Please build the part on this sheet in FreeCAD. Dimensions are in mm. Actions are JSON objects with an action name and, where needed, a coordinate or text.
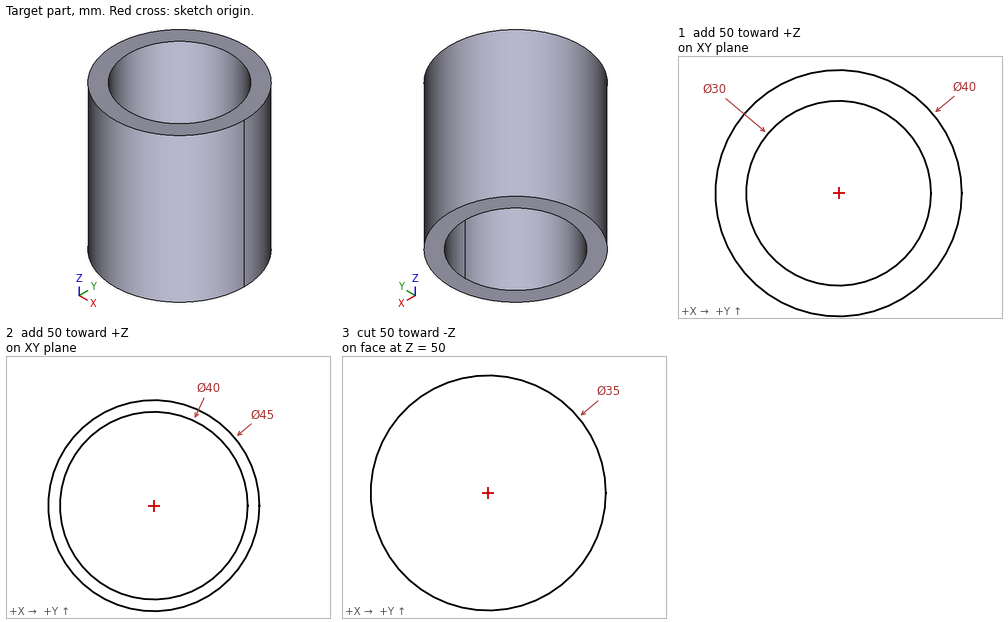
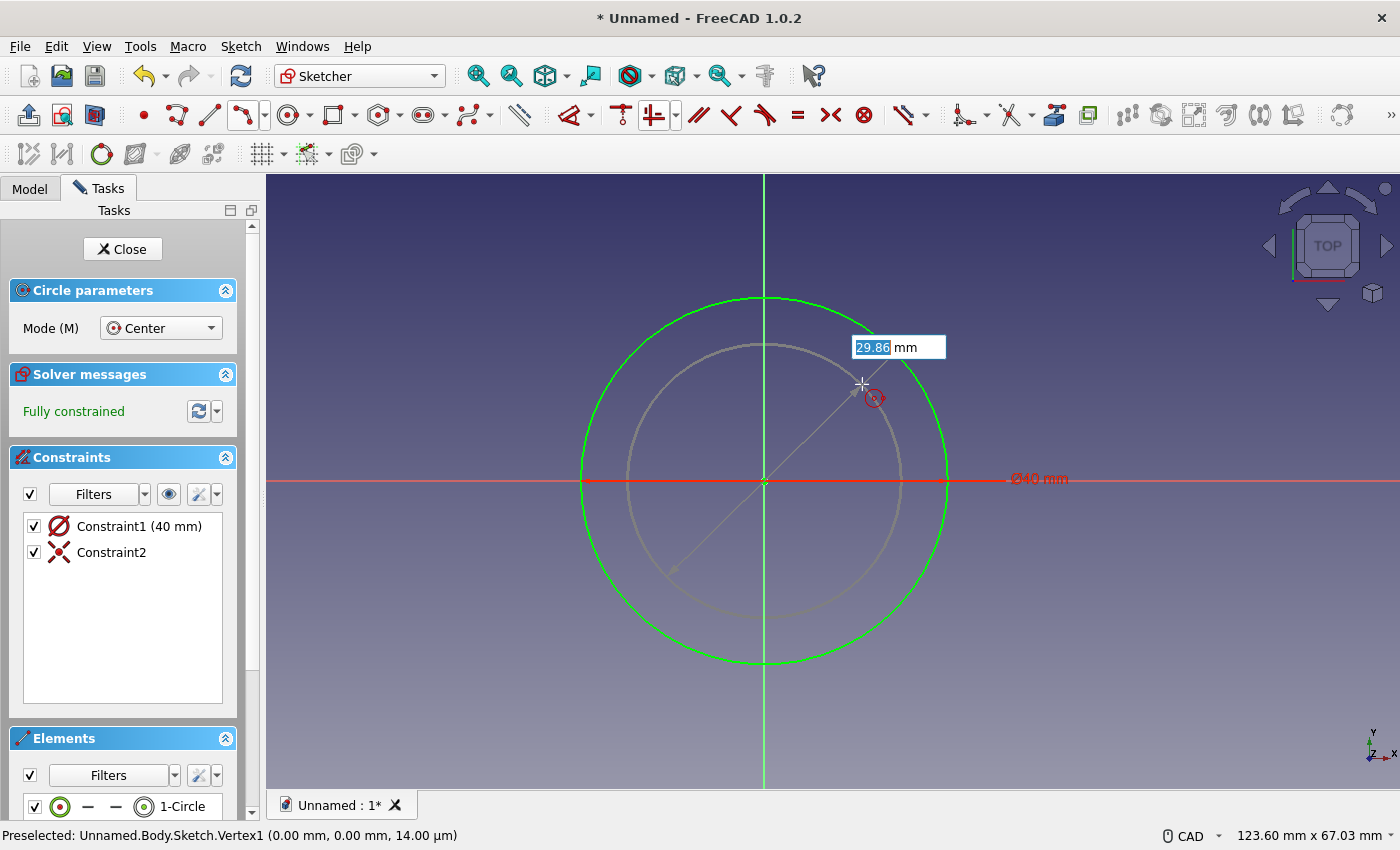
{"action": "type", "text": "30"}
{"action": "key", "text": "Return"}
{"action": "key", "text": "Escape"}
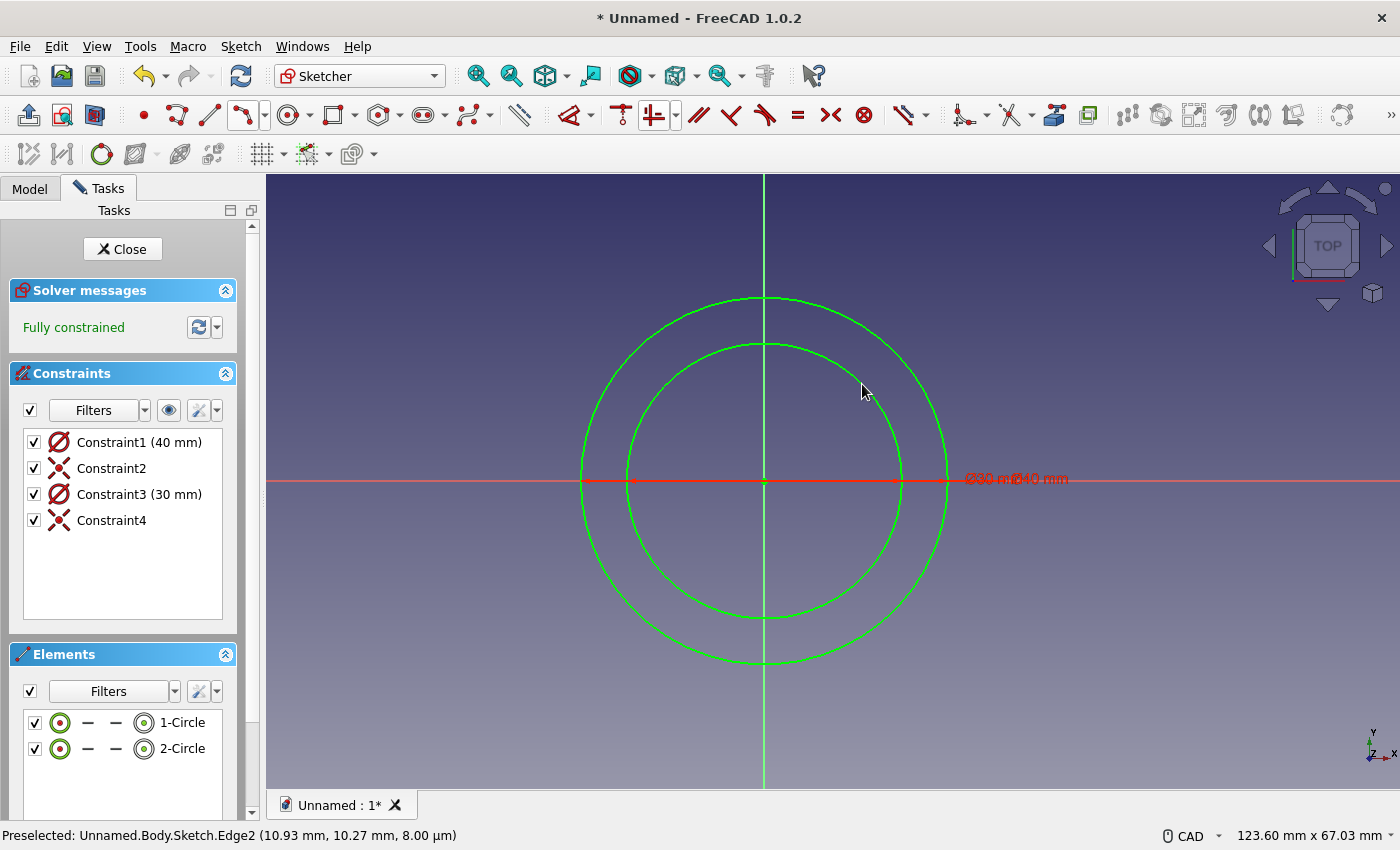
{"action": "left_click", "coordinate": [123, 249]}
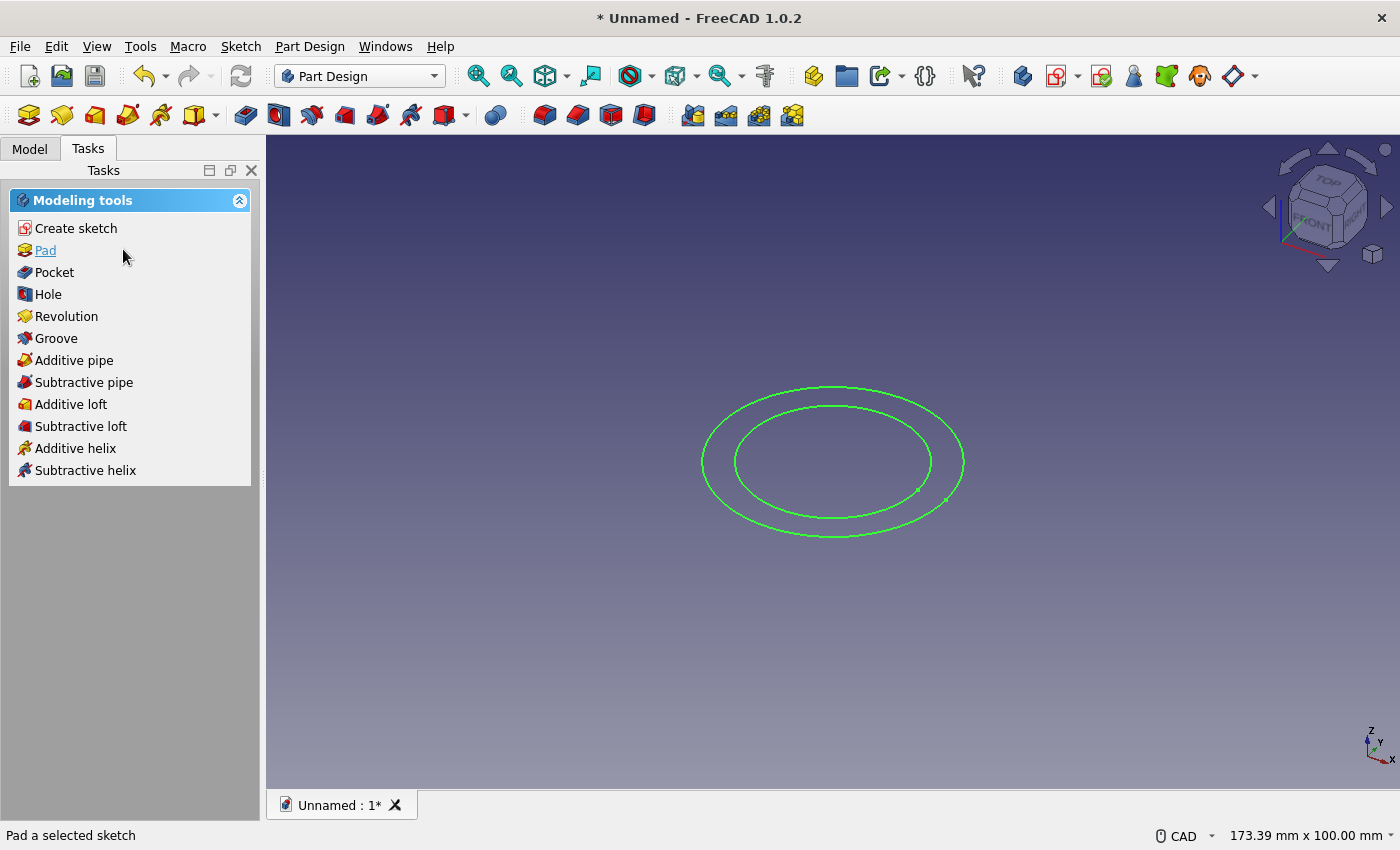
{"action": "left_click", "coordinate": [29, 116]}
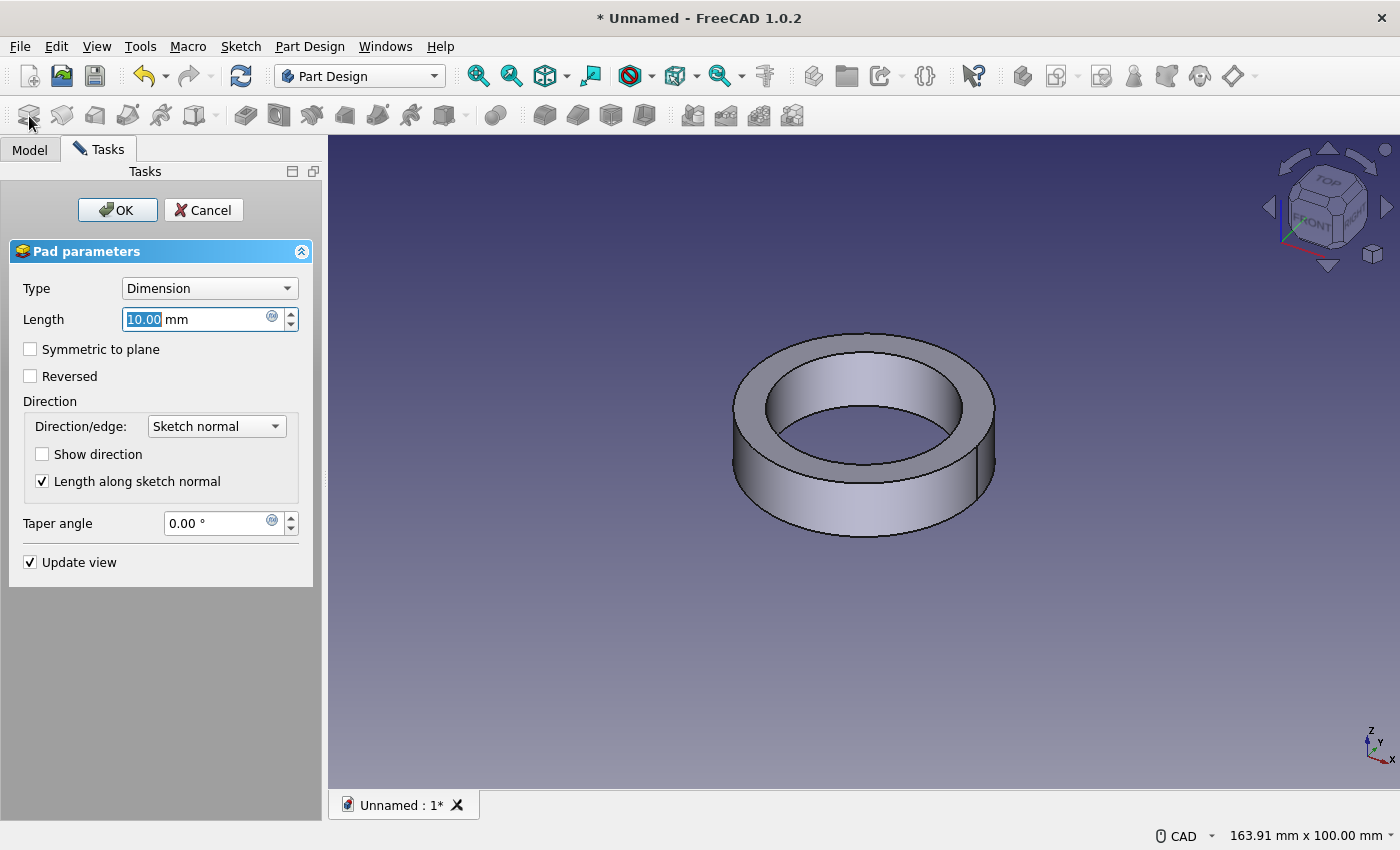
{"action": "type", "text": "50"}
{"action": "key", "text": "Tab"}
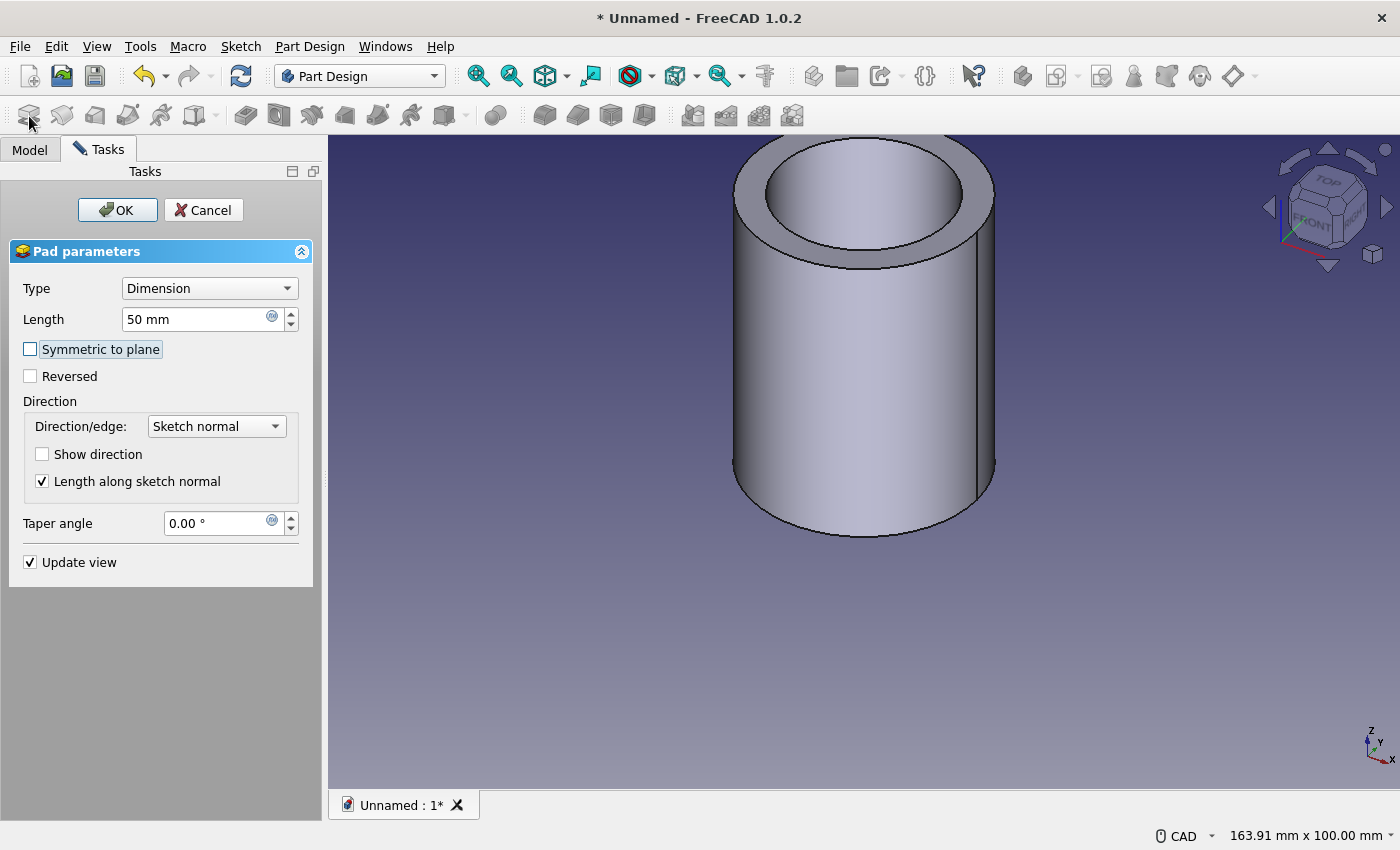
{"action": "left_click", "coordinate": [118, 210]}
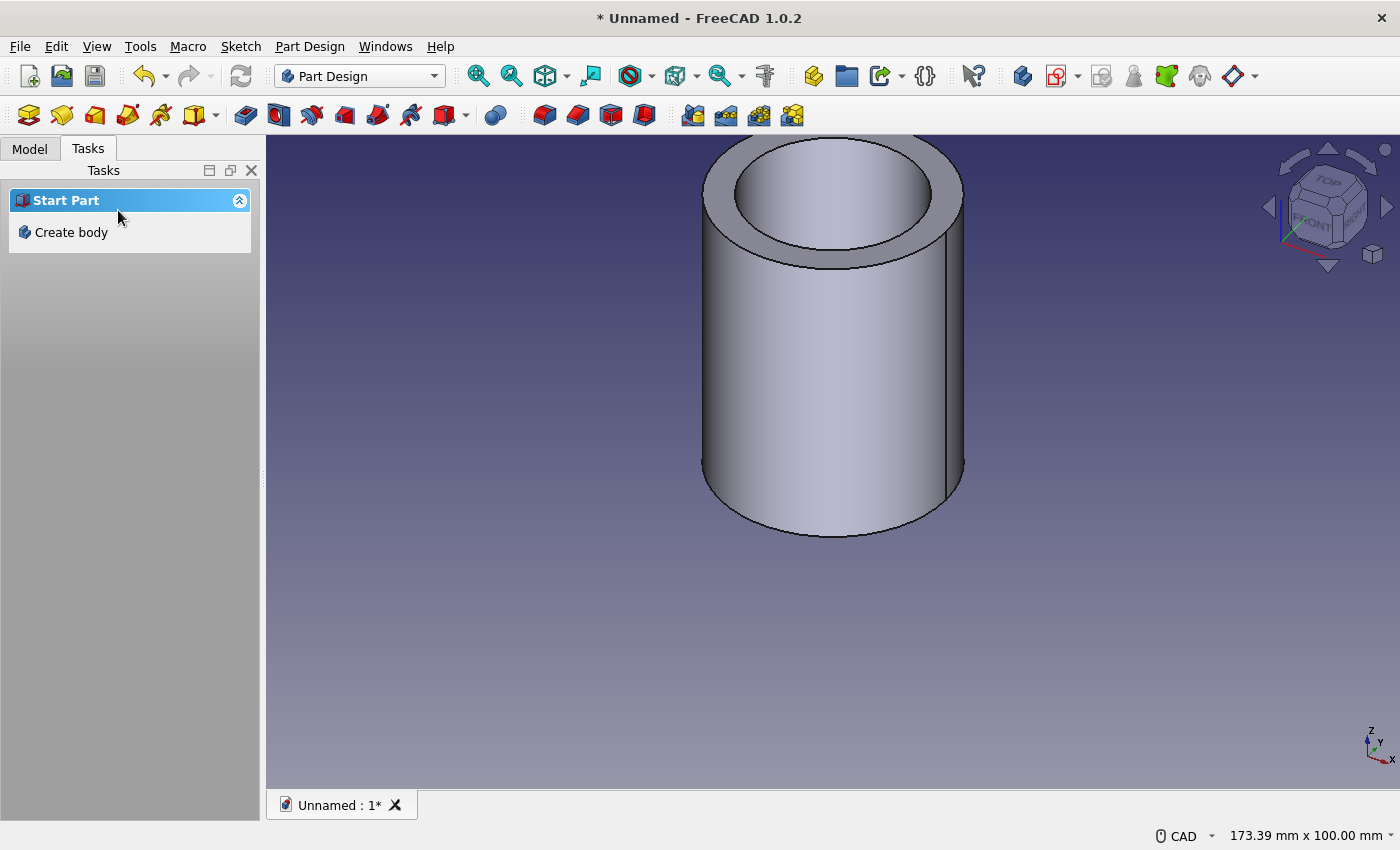
{"action": "key", "text": "v f"}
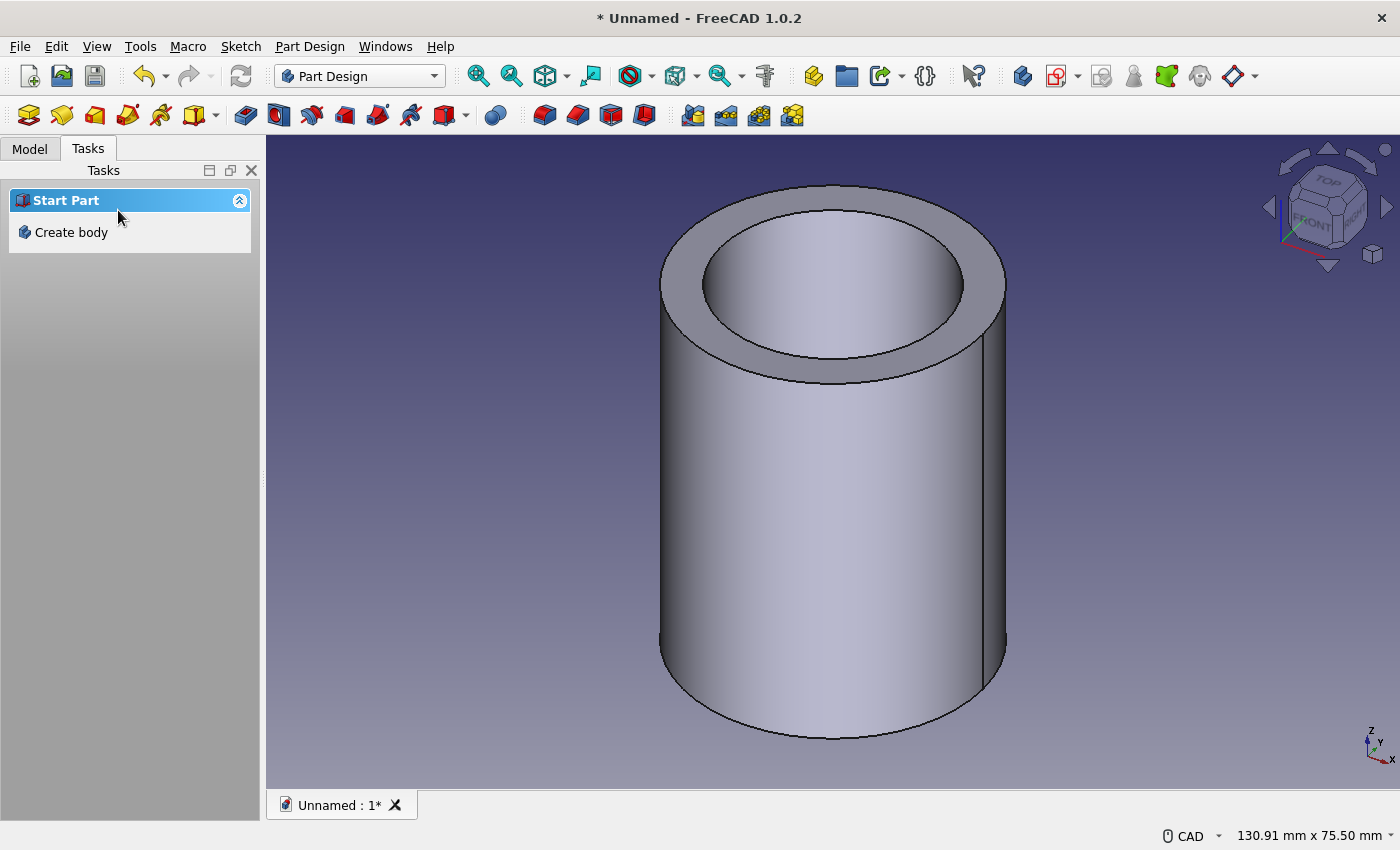
{"action": "left_click", "coordinate": [1056, 76]}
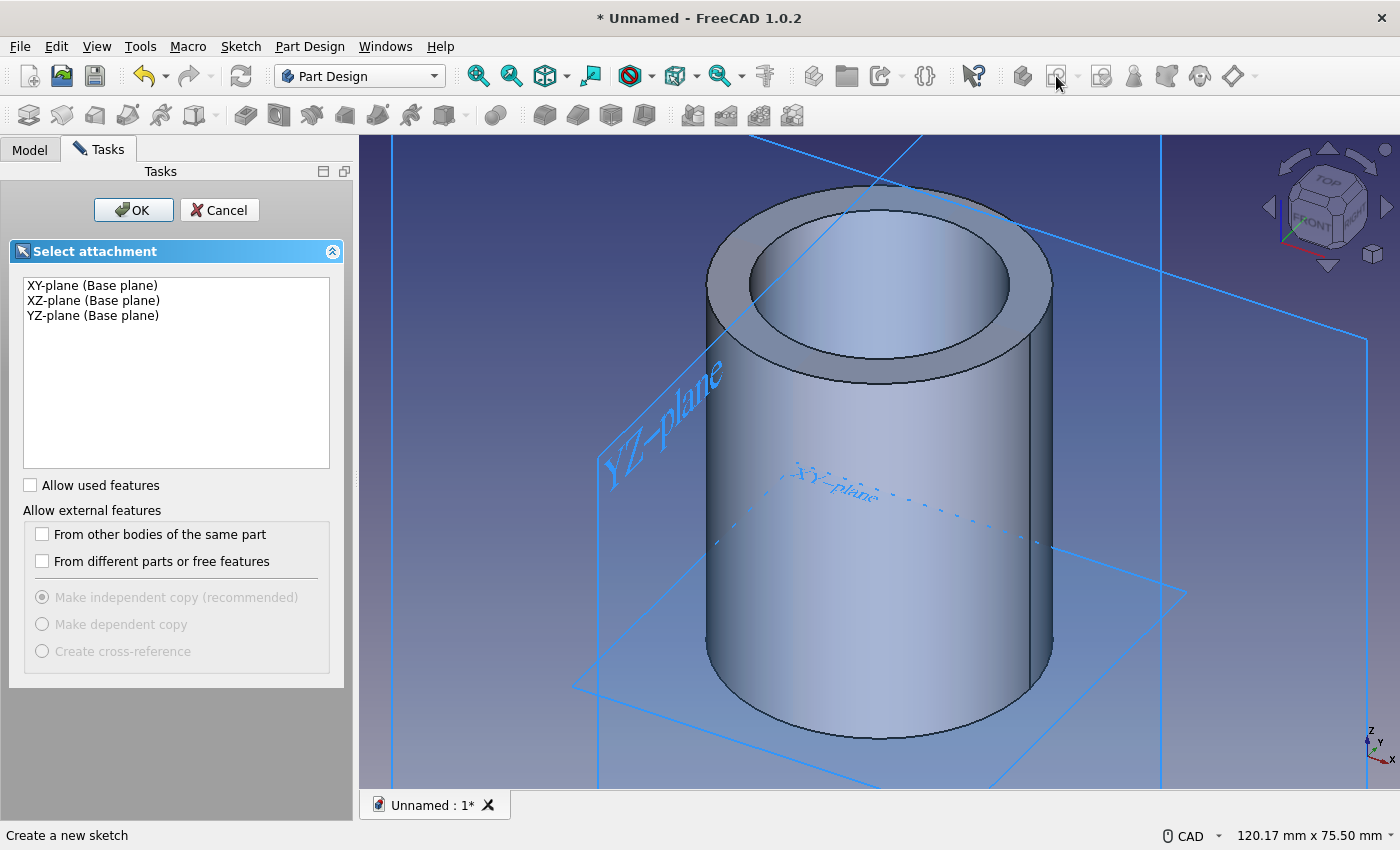
{"action": "left_click", "coordinate": [84, 286]}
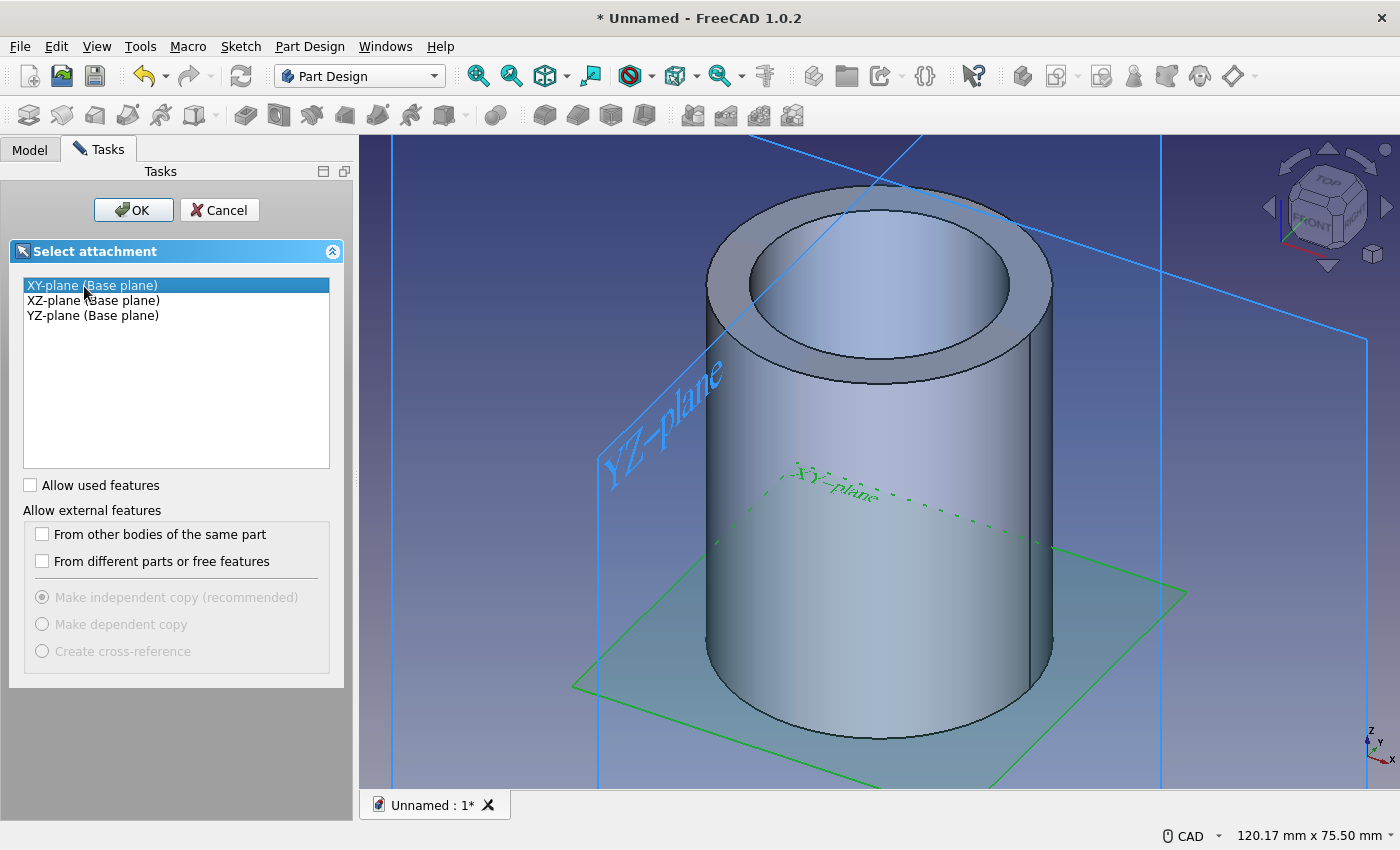
{"action": "left_click", "coordinate": [134, 210]}